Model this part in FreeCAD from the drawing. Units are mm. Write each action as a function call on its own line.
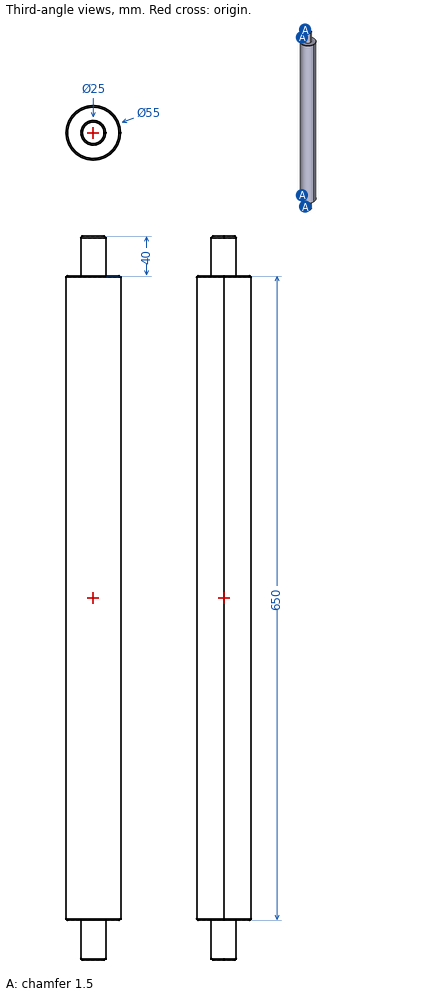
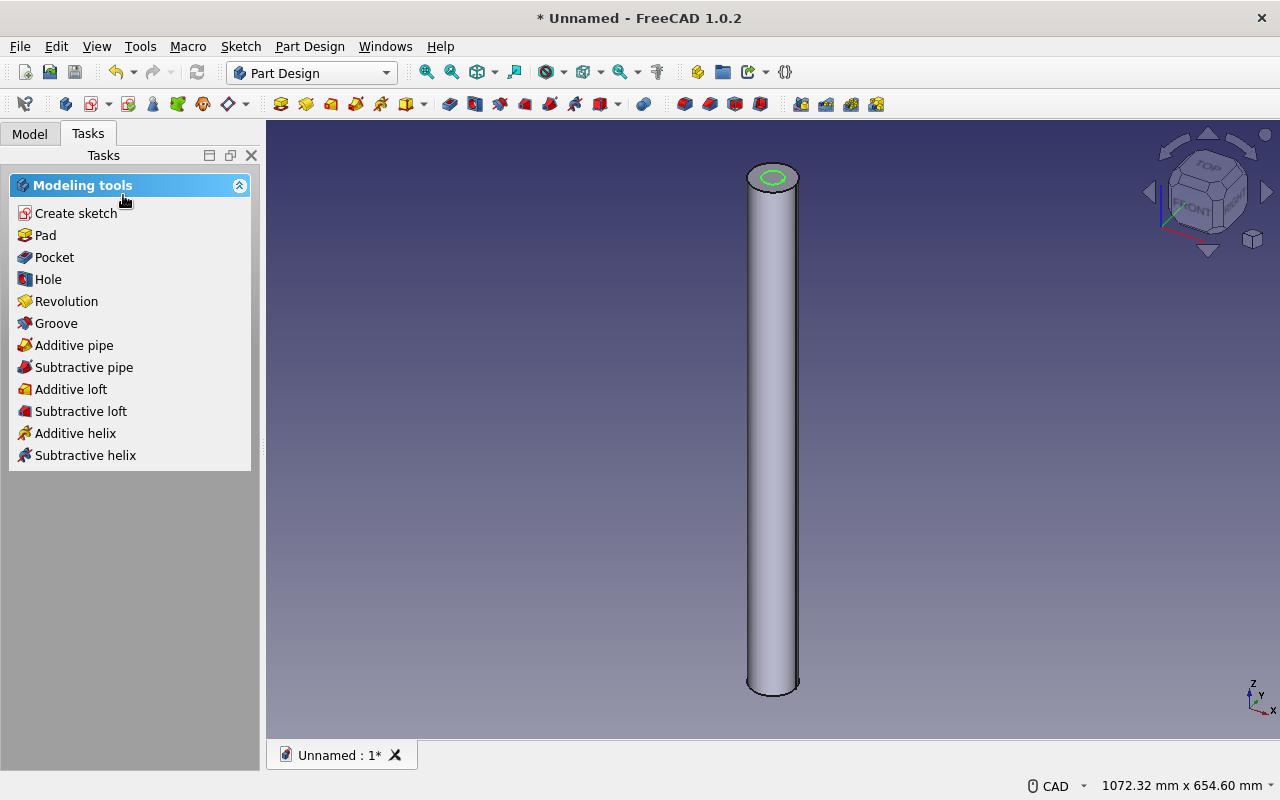
click(281, 104)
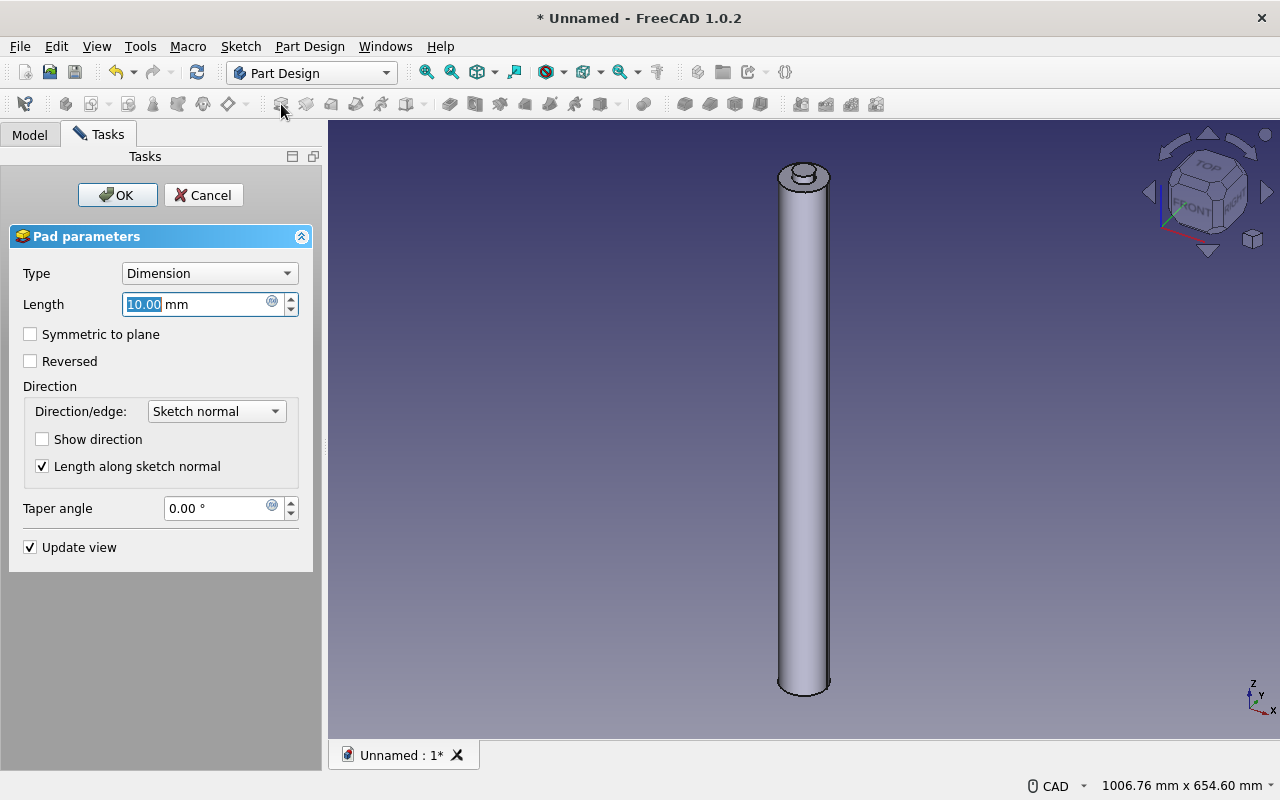
text(40)
key(Tab)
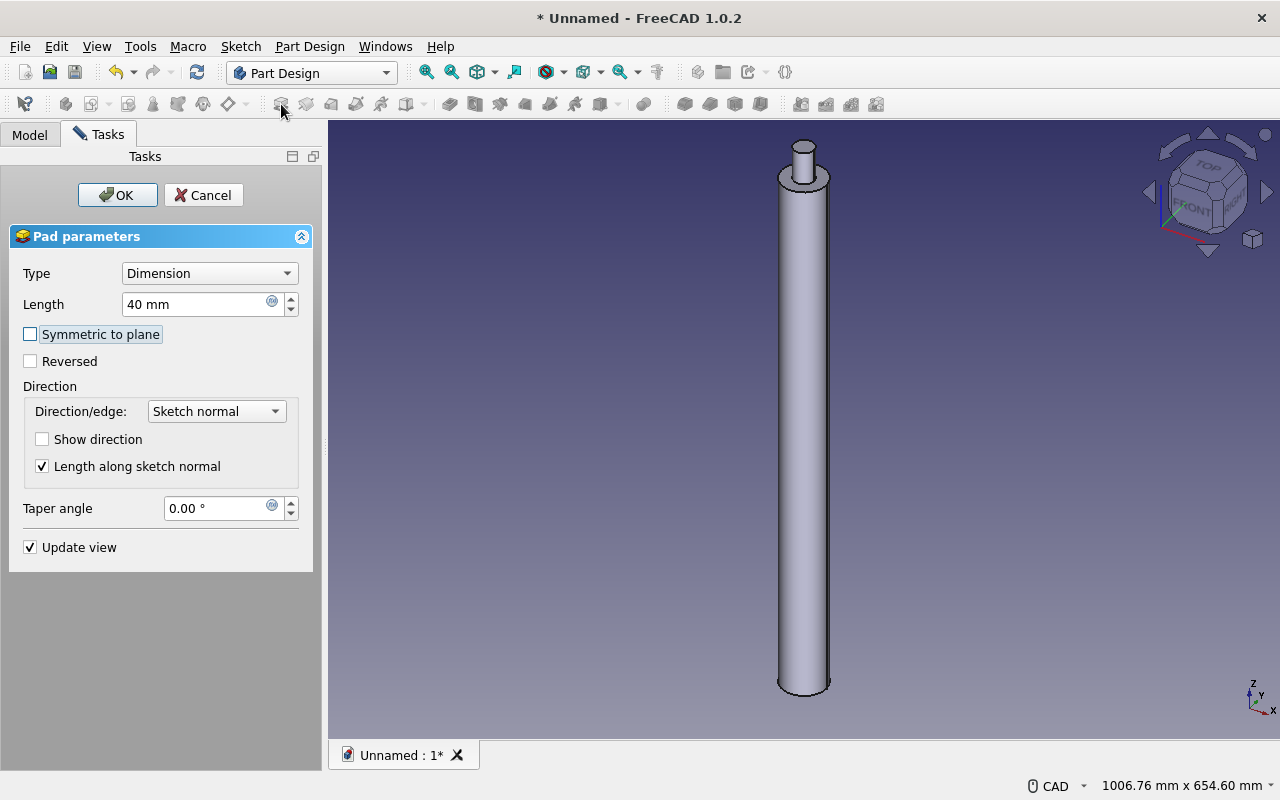
click(118, 195)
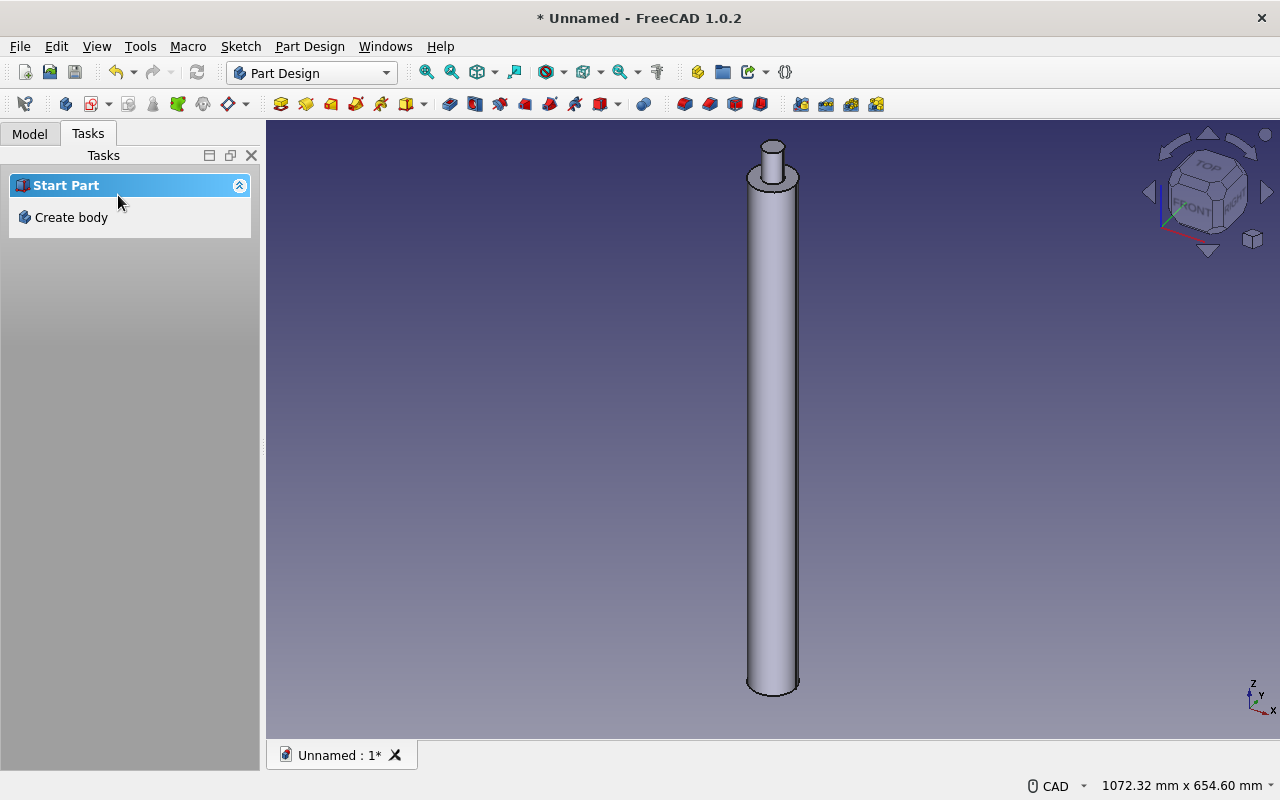
click(30, 134)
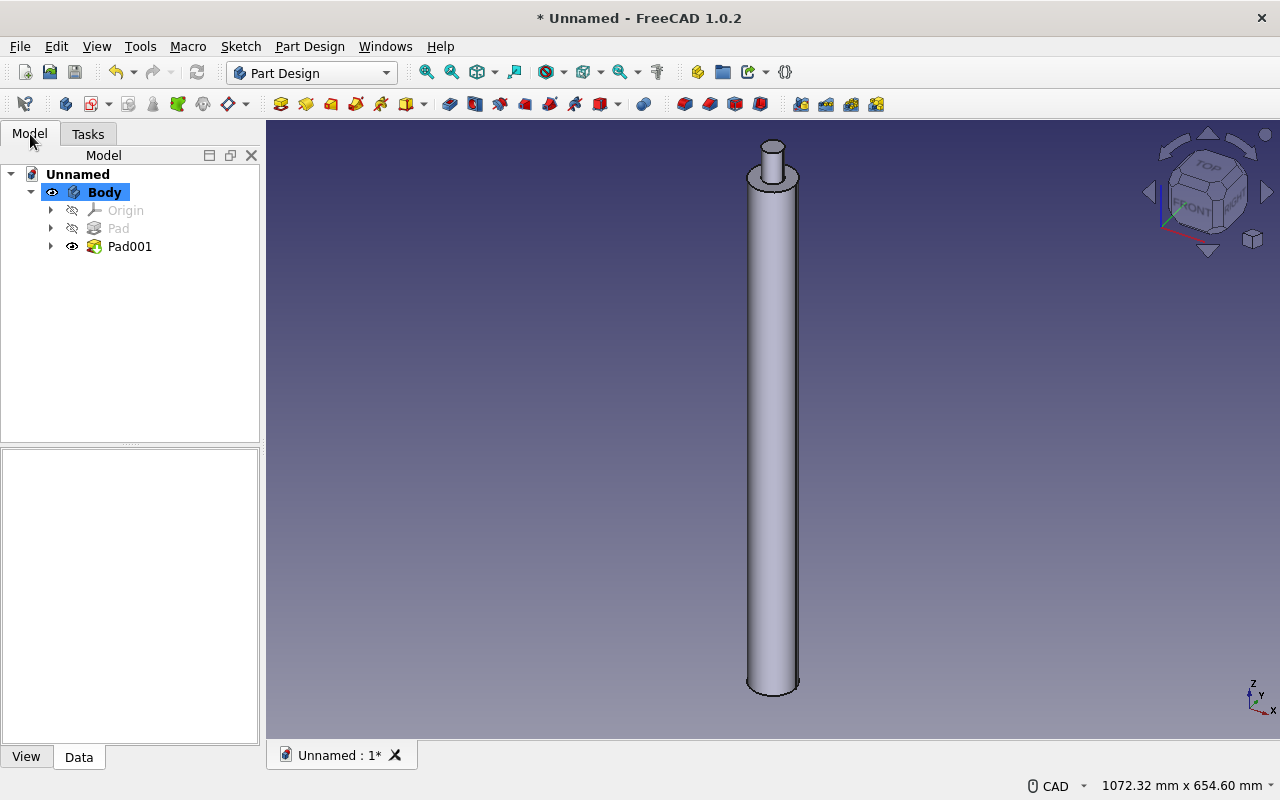
click(117, 246)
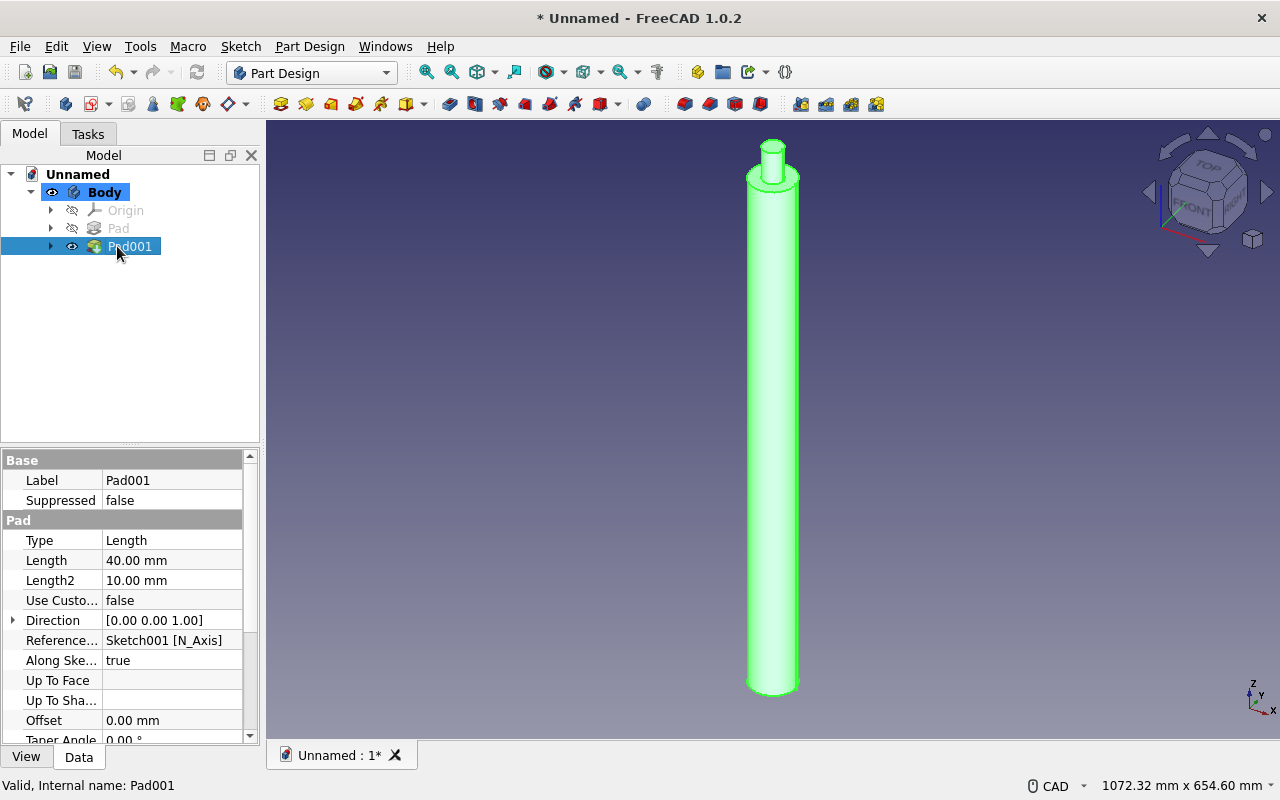
click(801, 104)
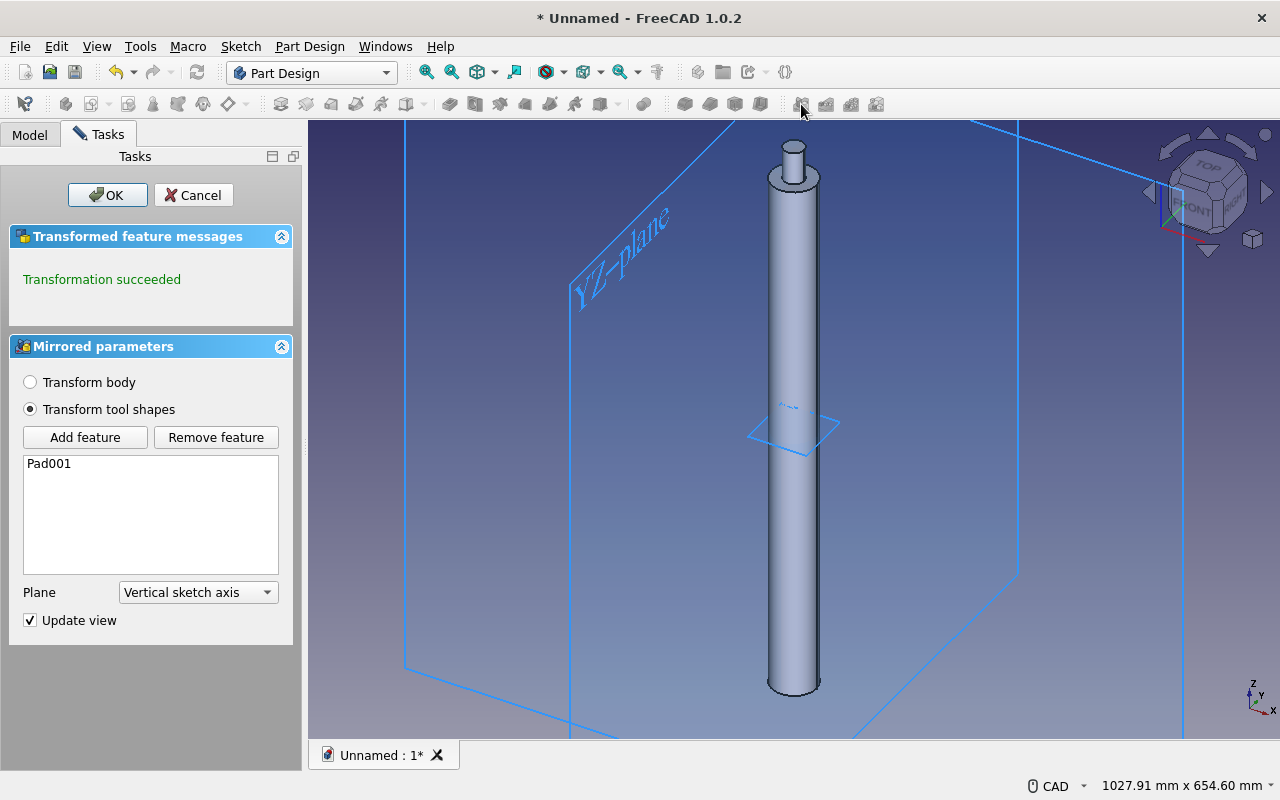
click(199, 592)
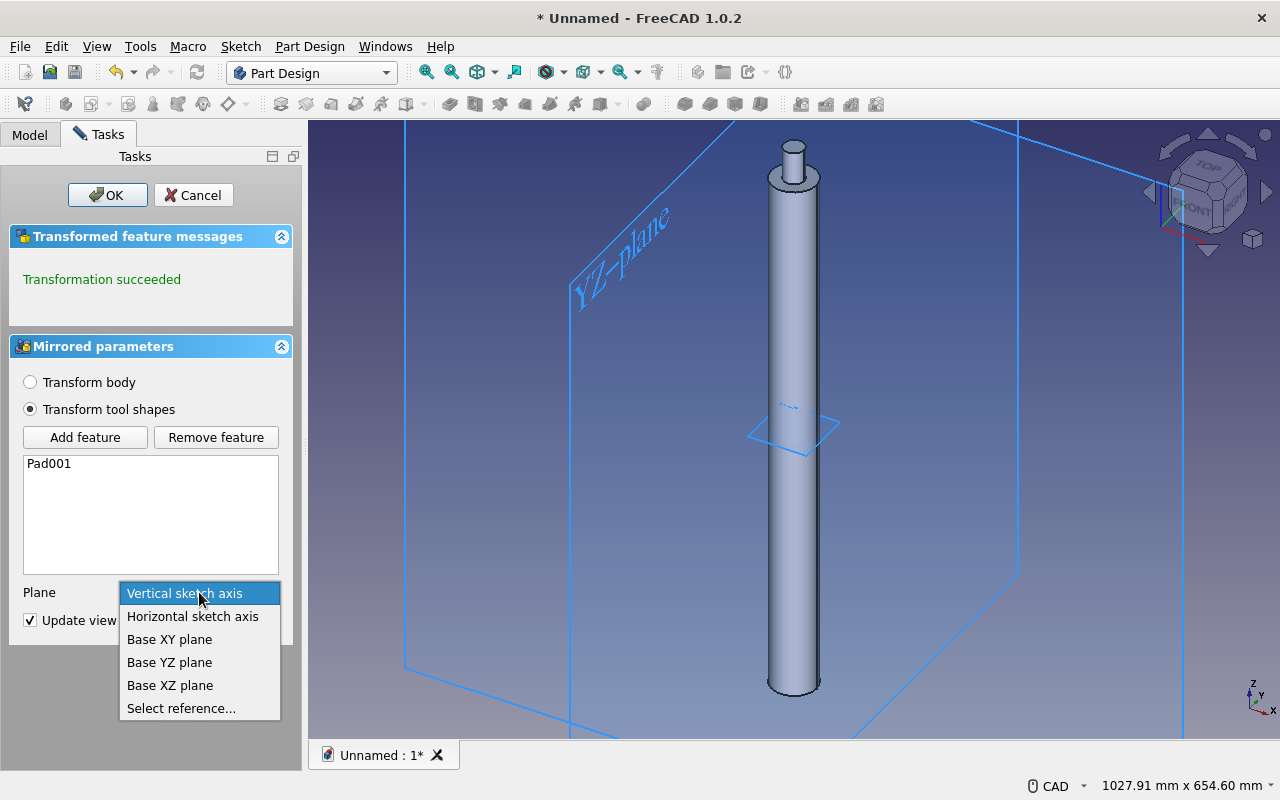
click(198, 640)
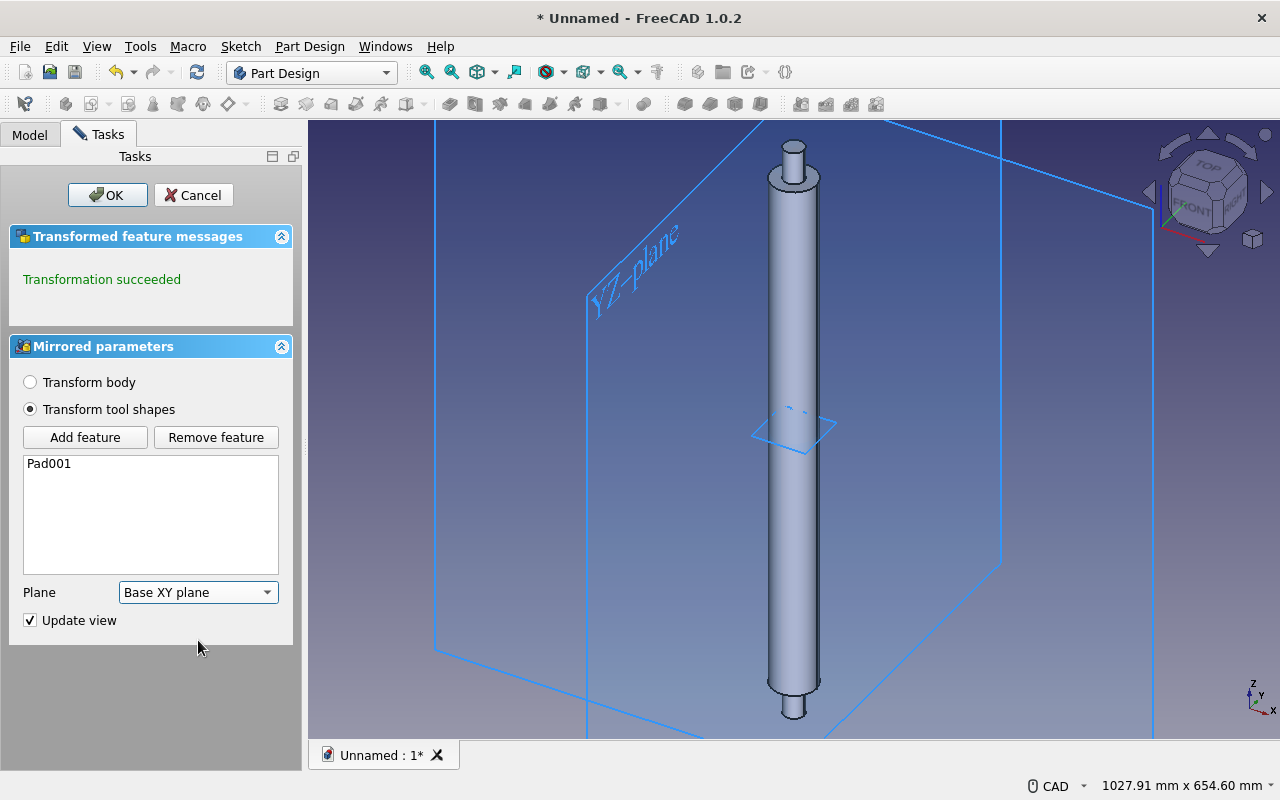
click(108, 195)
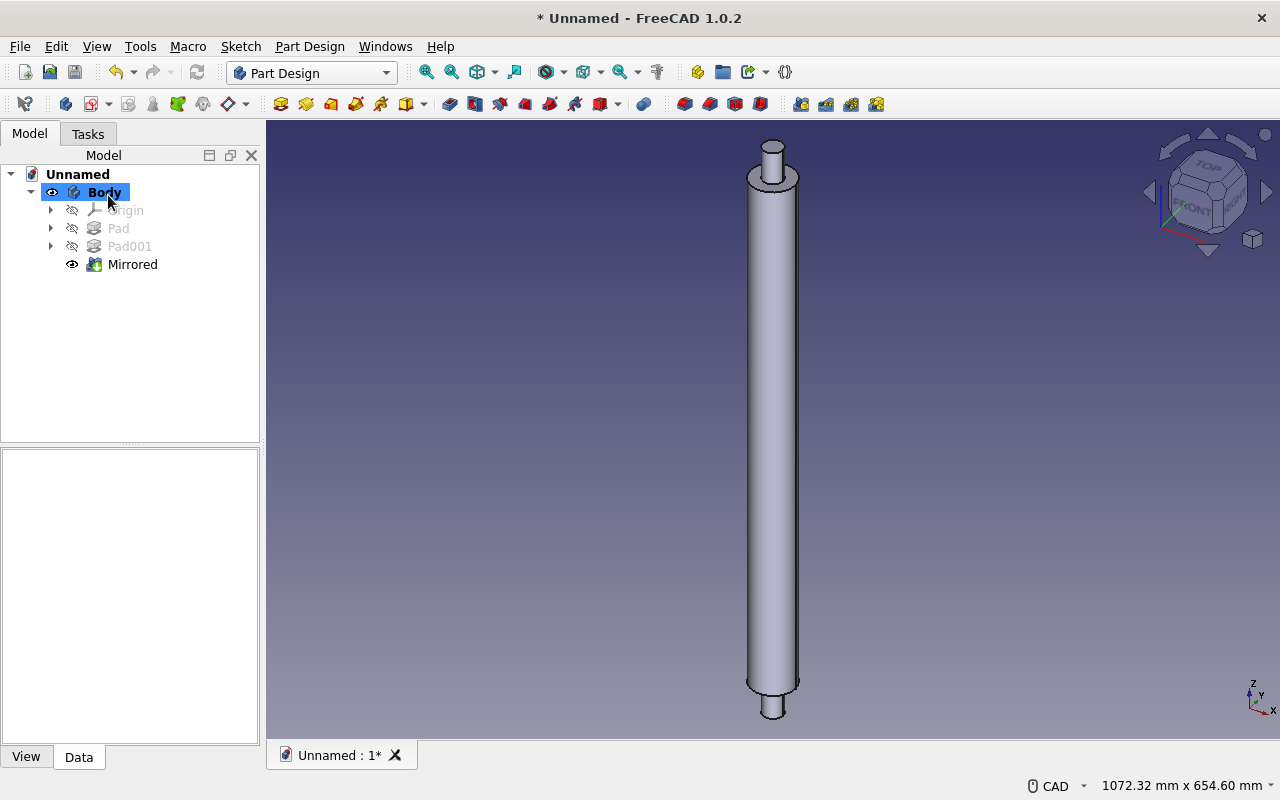
click(747, 178)